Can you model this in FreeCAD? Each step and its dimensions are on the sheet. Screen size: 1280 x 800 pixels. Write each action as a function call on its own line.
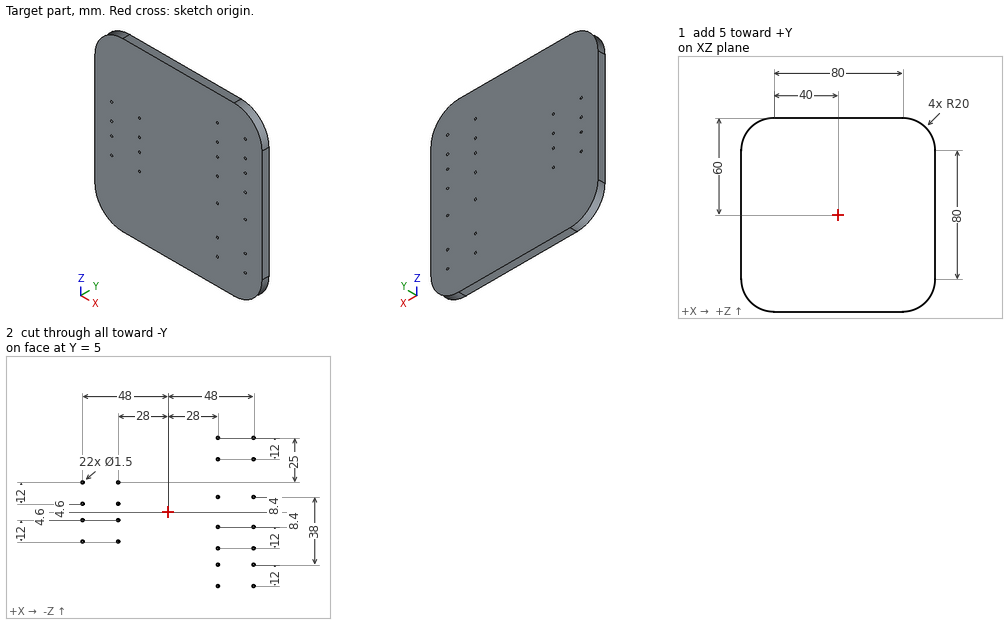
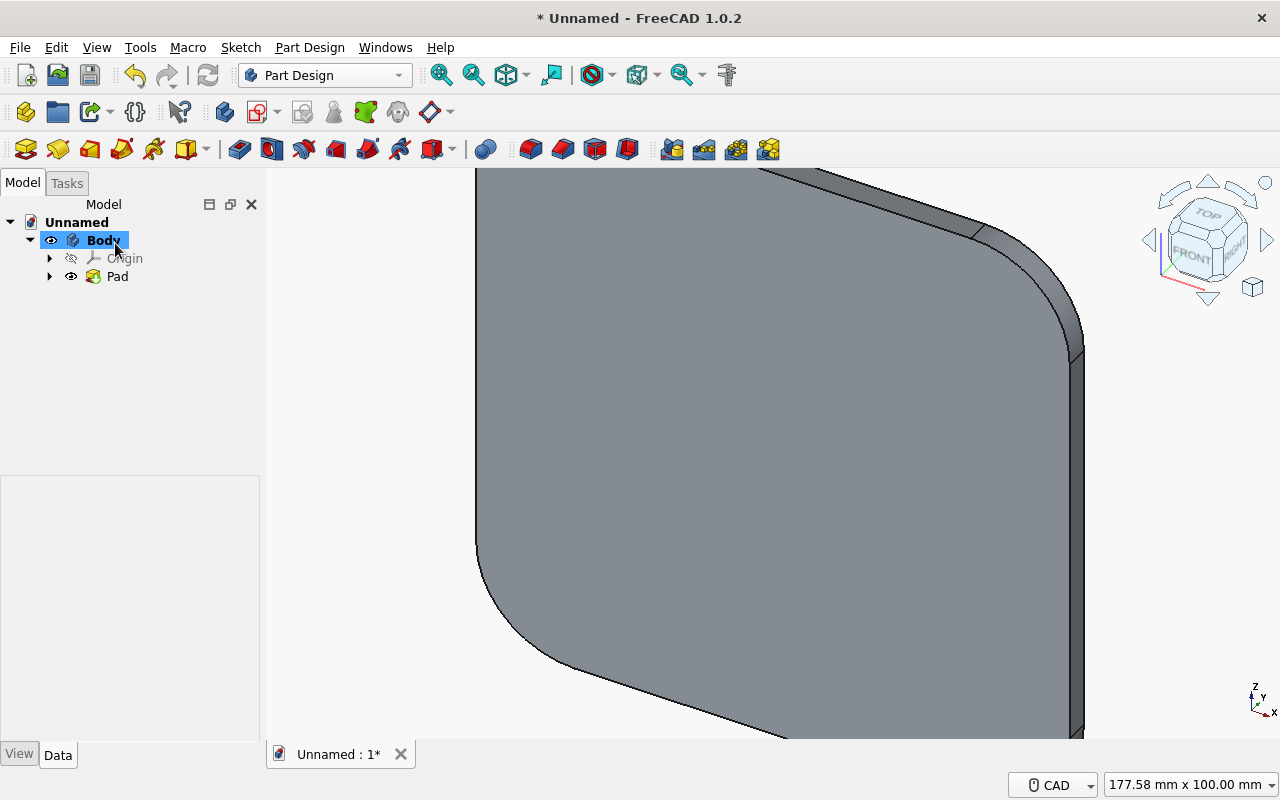
click(442, 76)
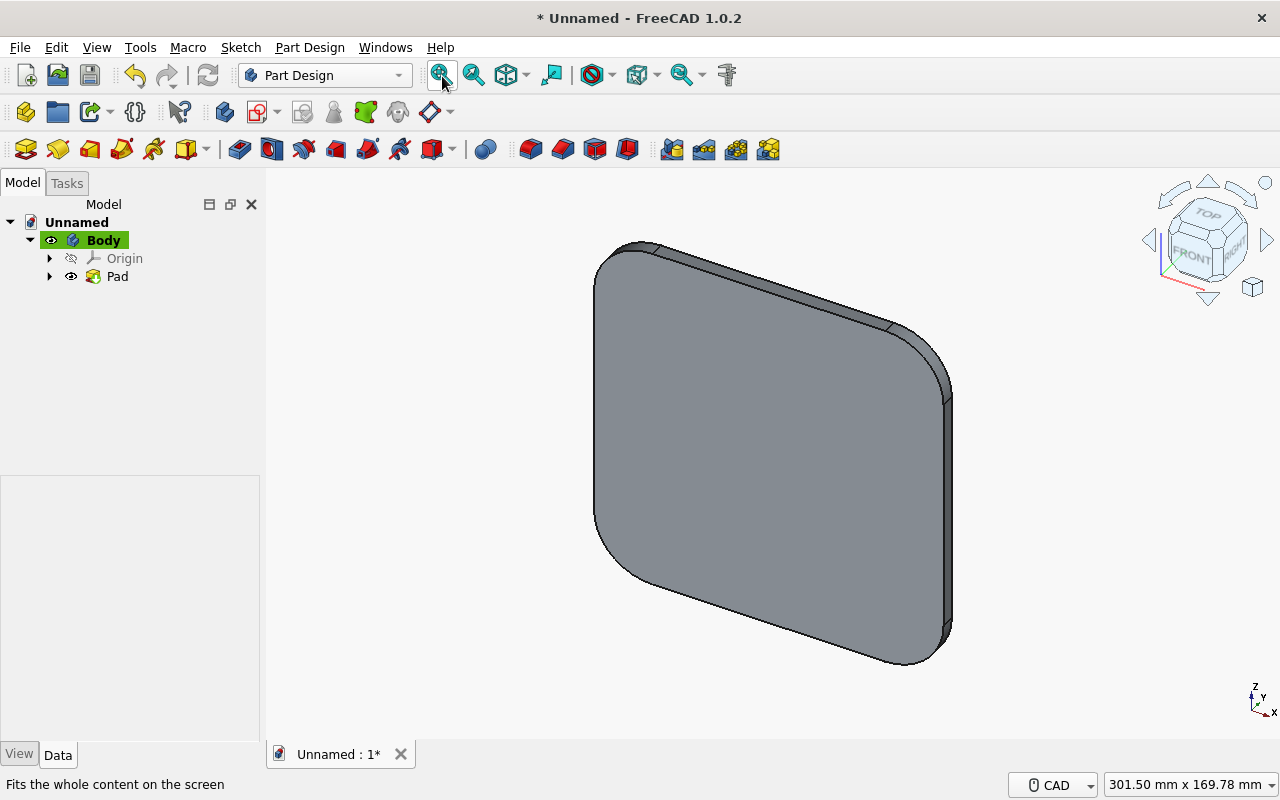
key(4)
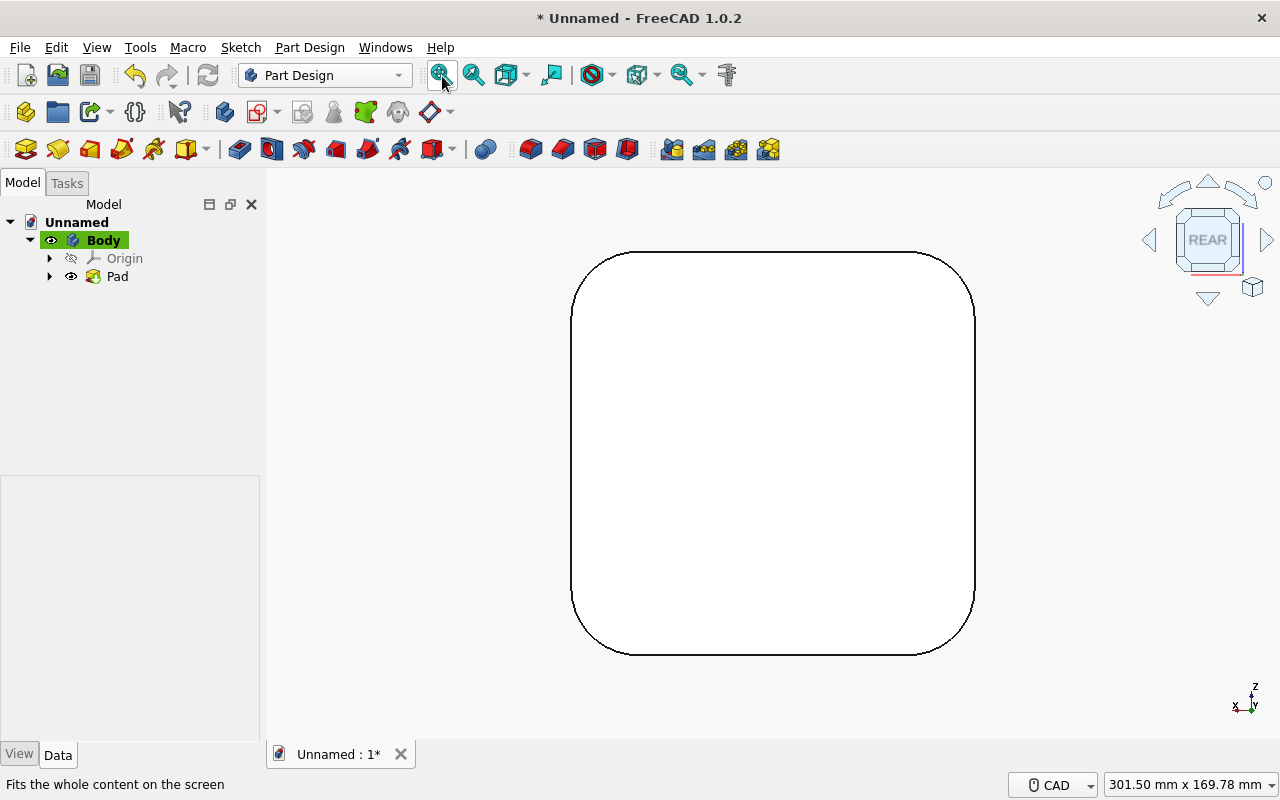
click(773, 452)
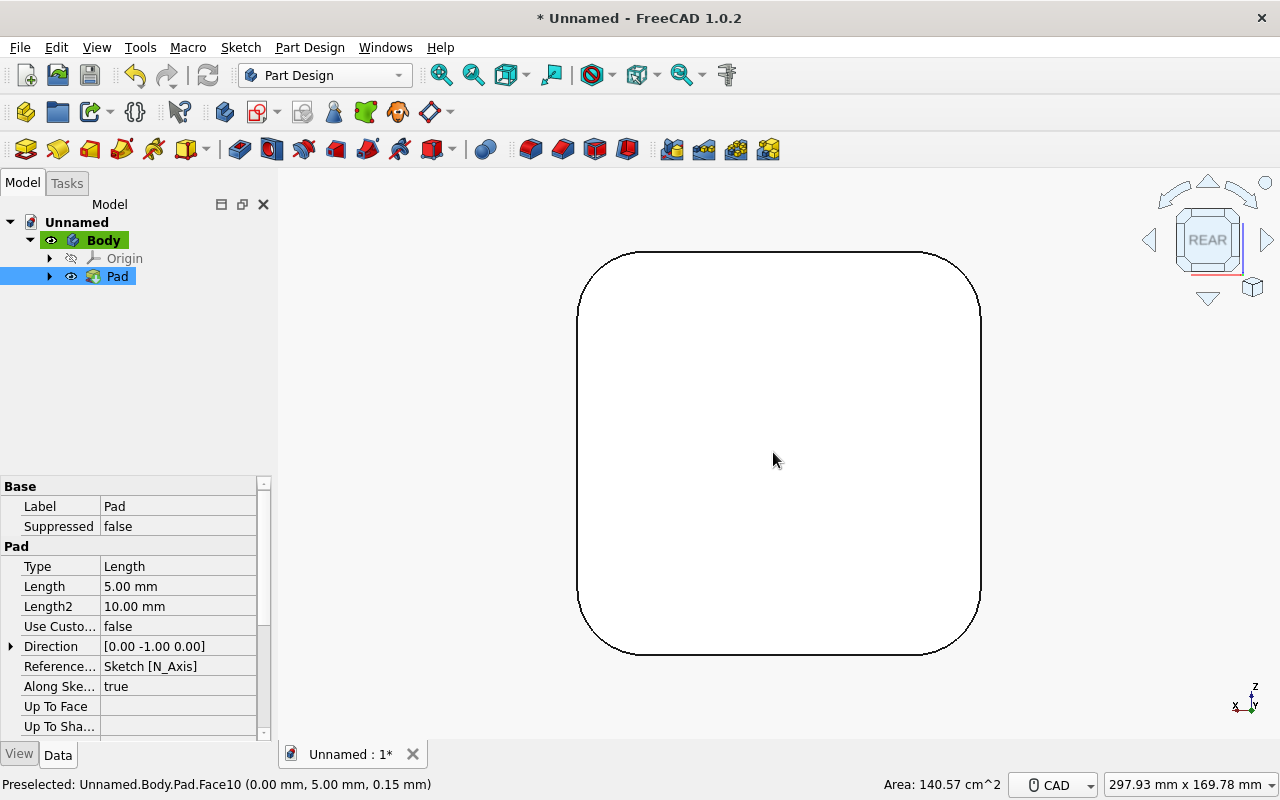
click(258, 112)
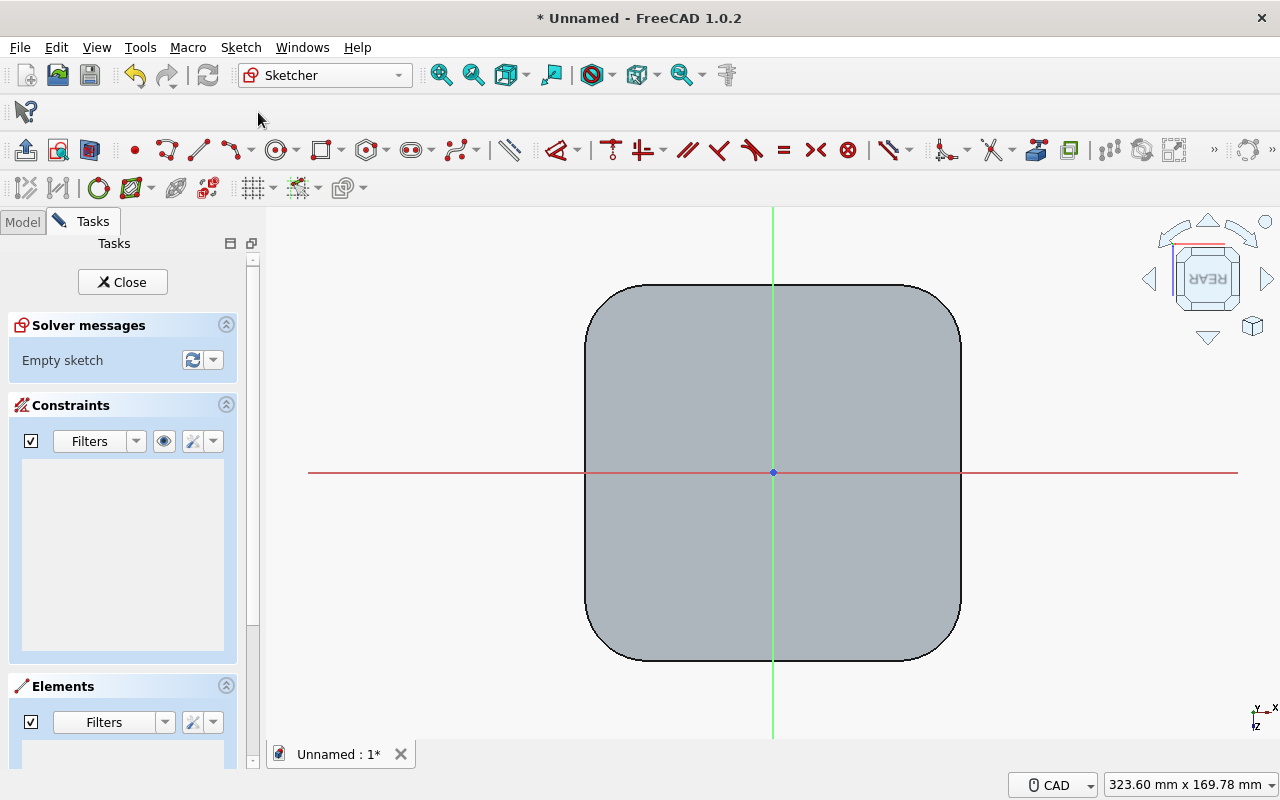
click(276, 150)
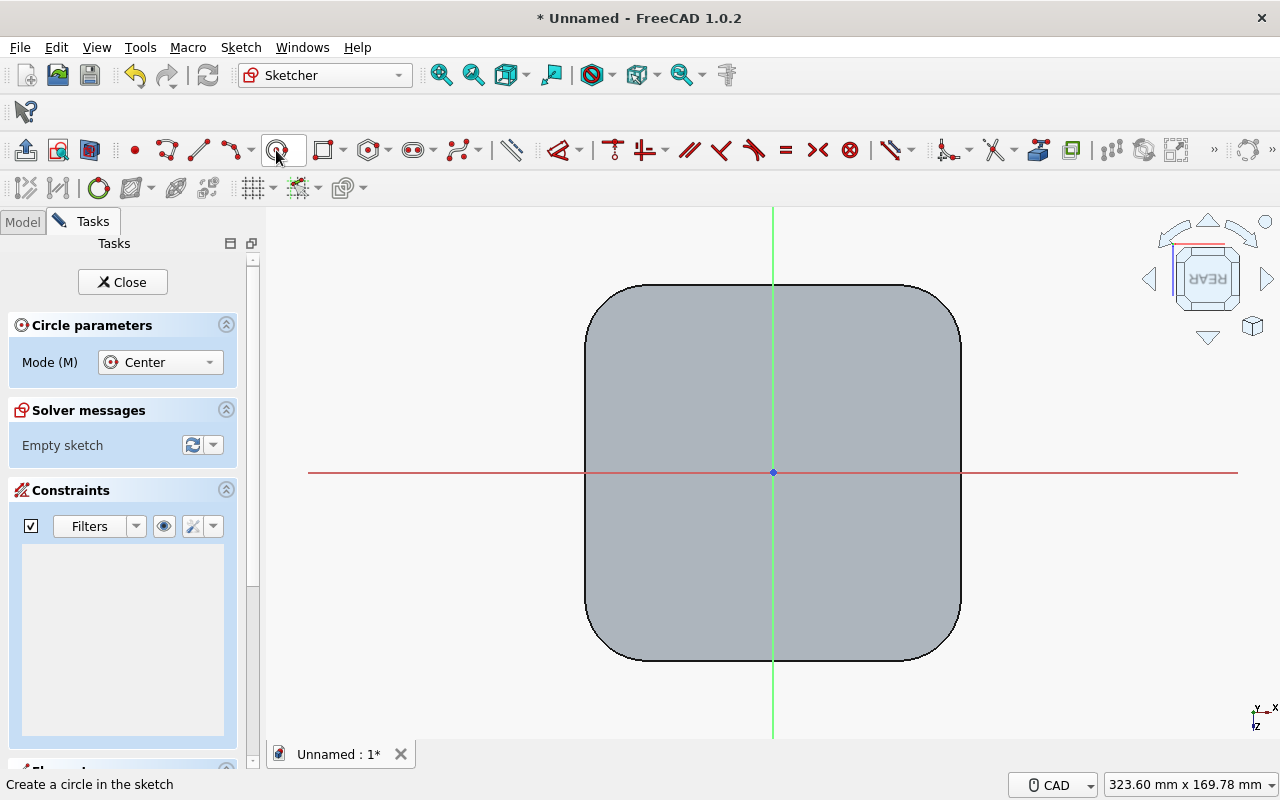
scroll(623, 421, up, 12)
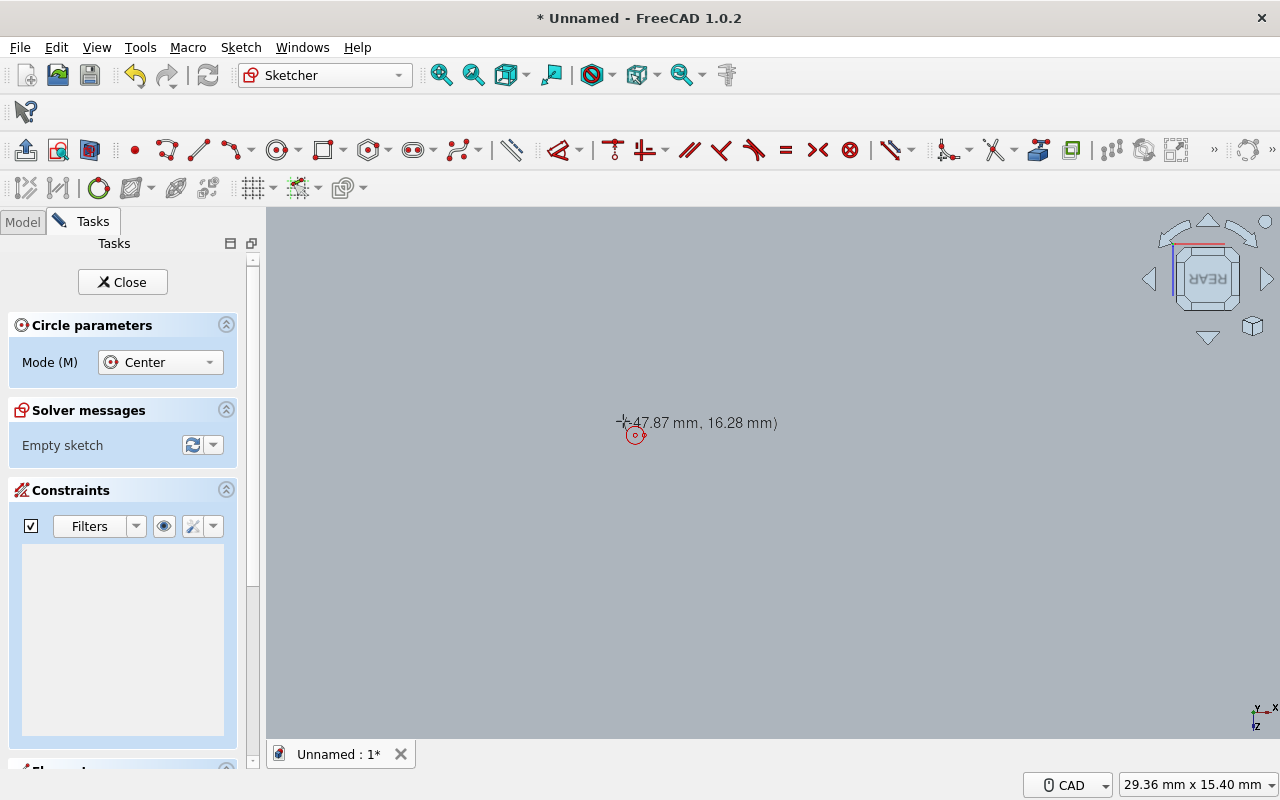
scroll(509, 409, down, 11)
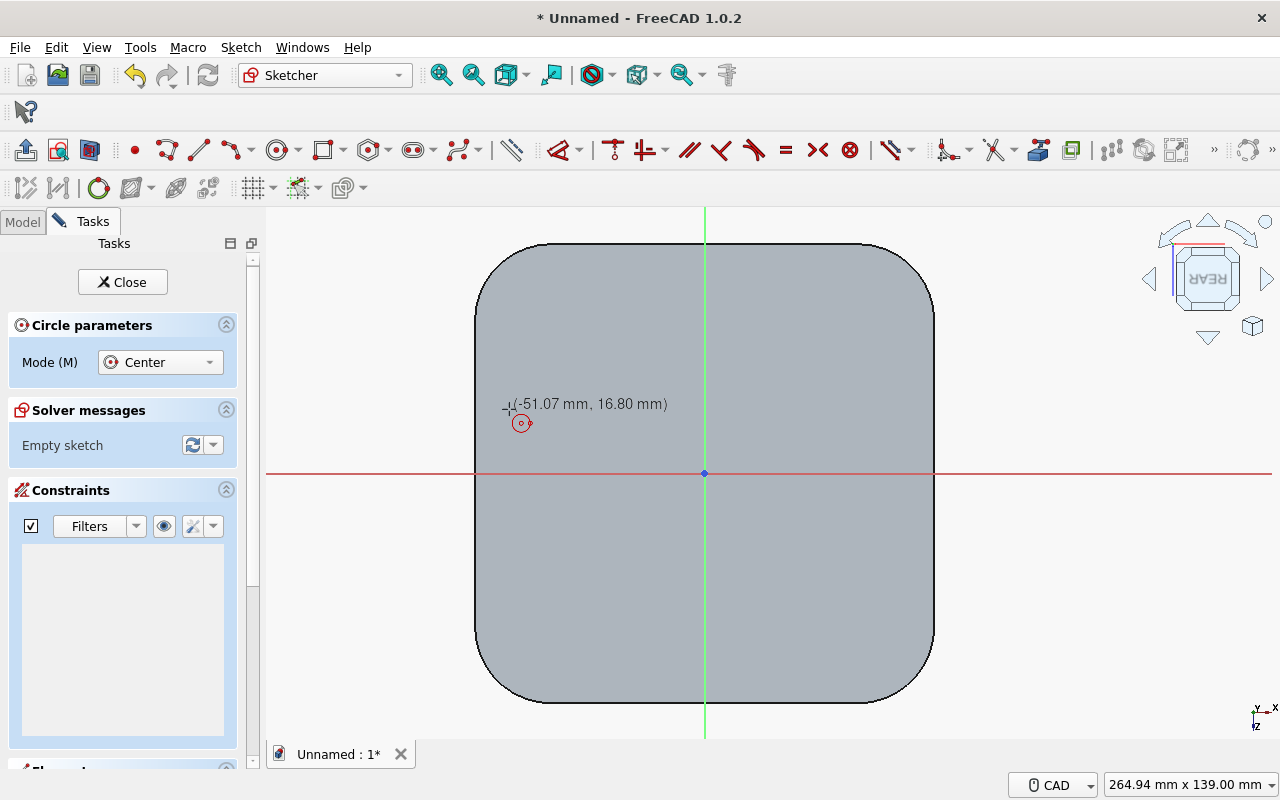
click(521, 410)
move(523, 408)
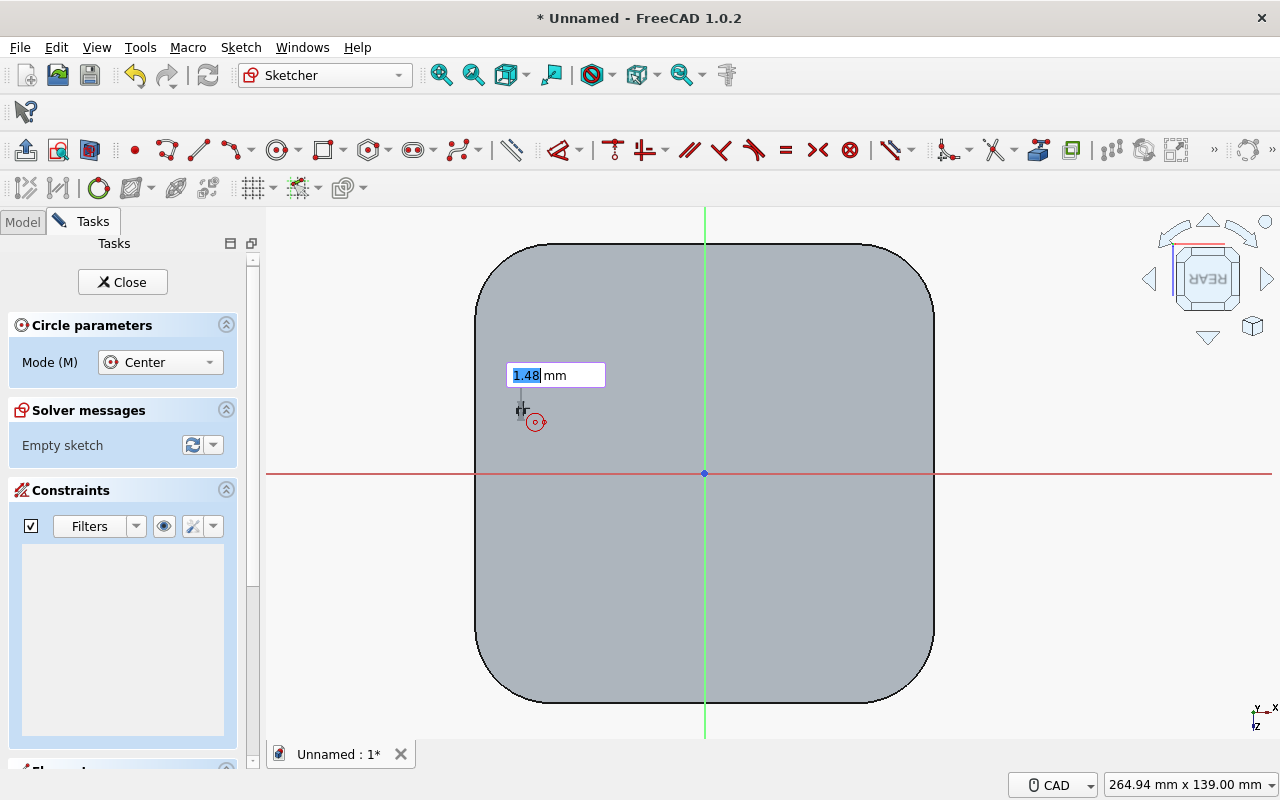
text(1.5)
key(Return)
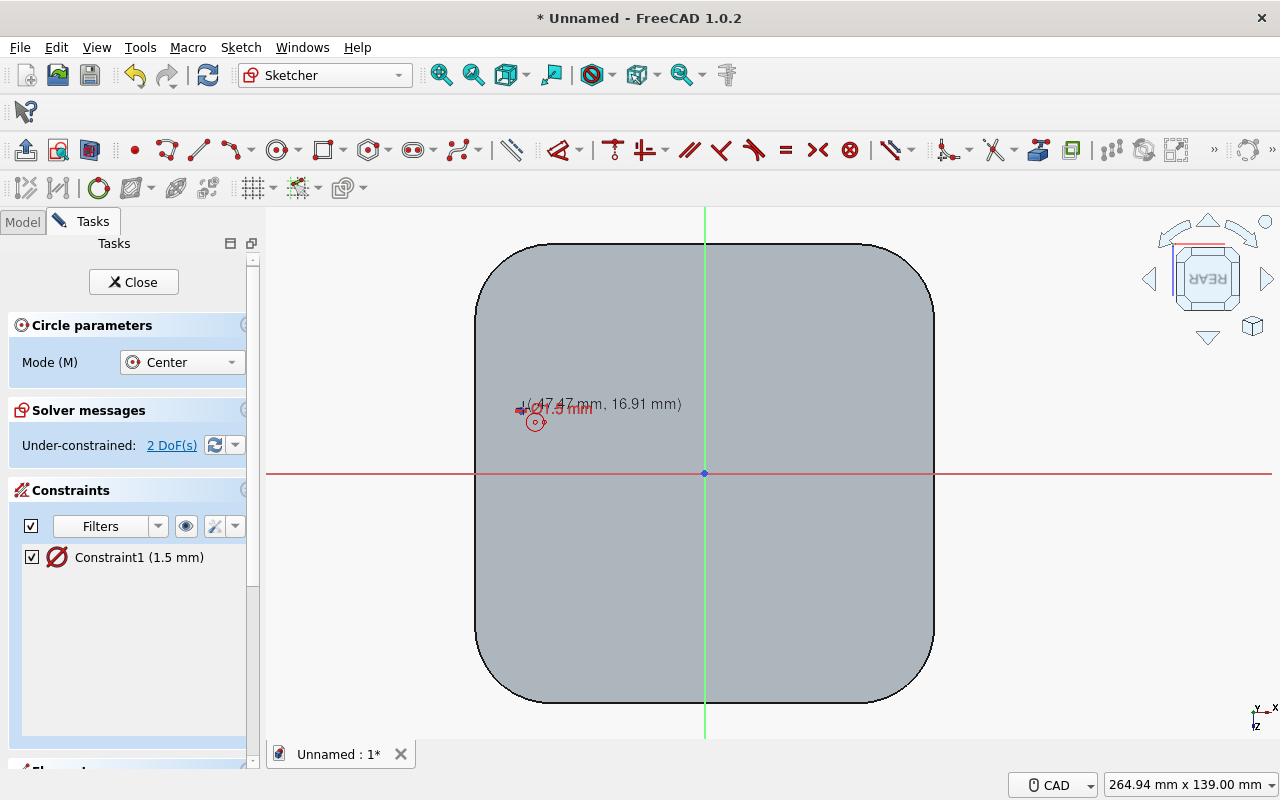
scroll(598, 410, up, 11)